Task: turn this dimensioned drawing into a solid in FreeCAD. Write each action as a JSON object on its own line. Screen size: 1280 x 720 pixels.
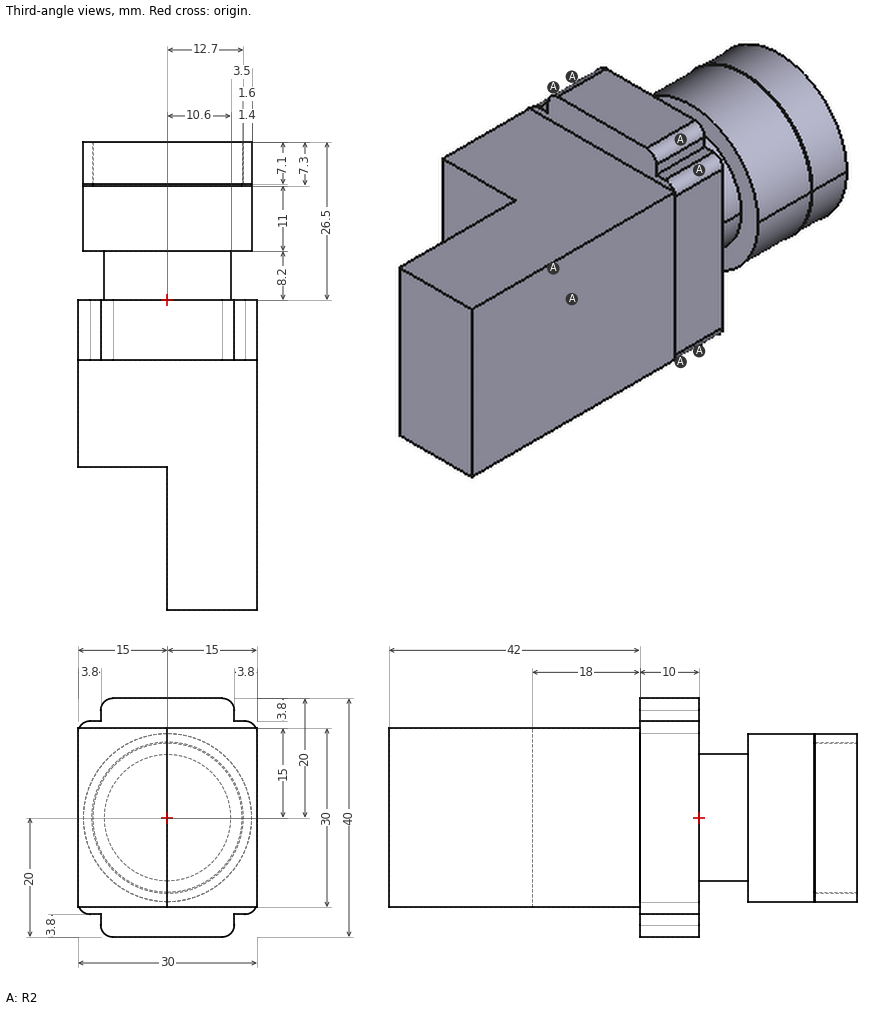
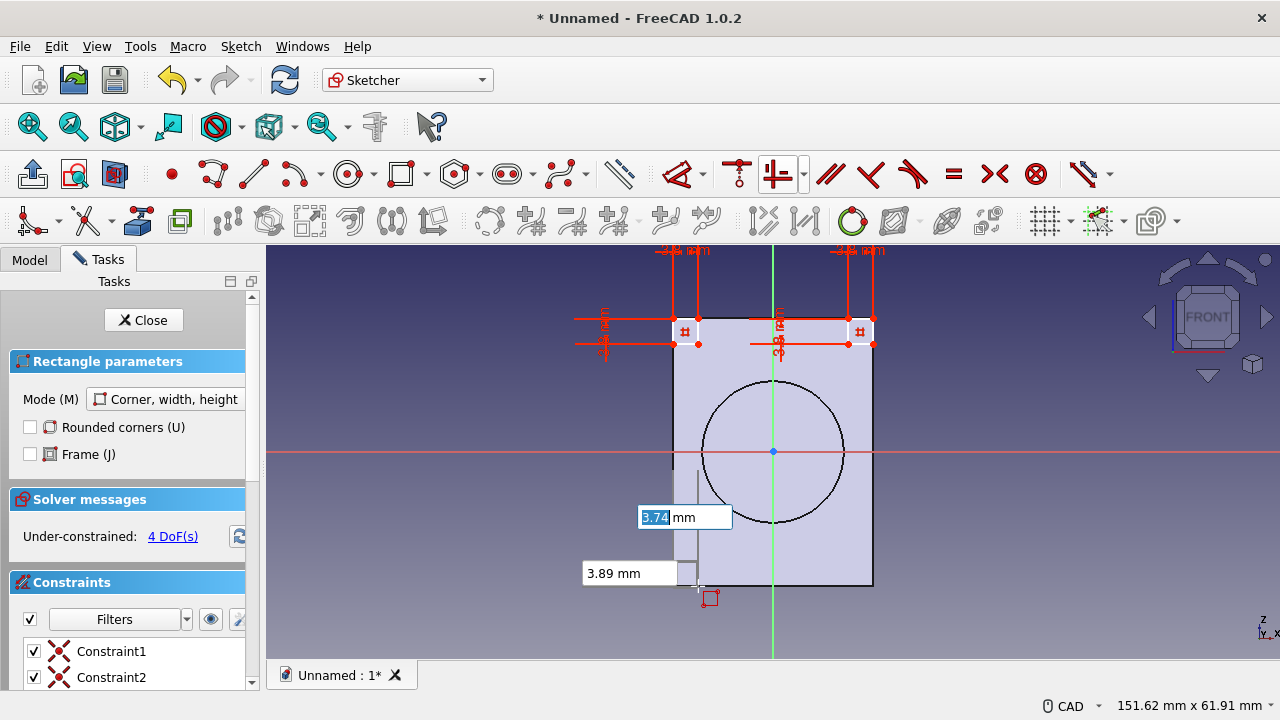
{"action": "type", "text": "3.8"}
{"action": "key", "text": "Tab"}
{"action": "type", "text": "3.8"}
{"action": "key", "text": "Return"}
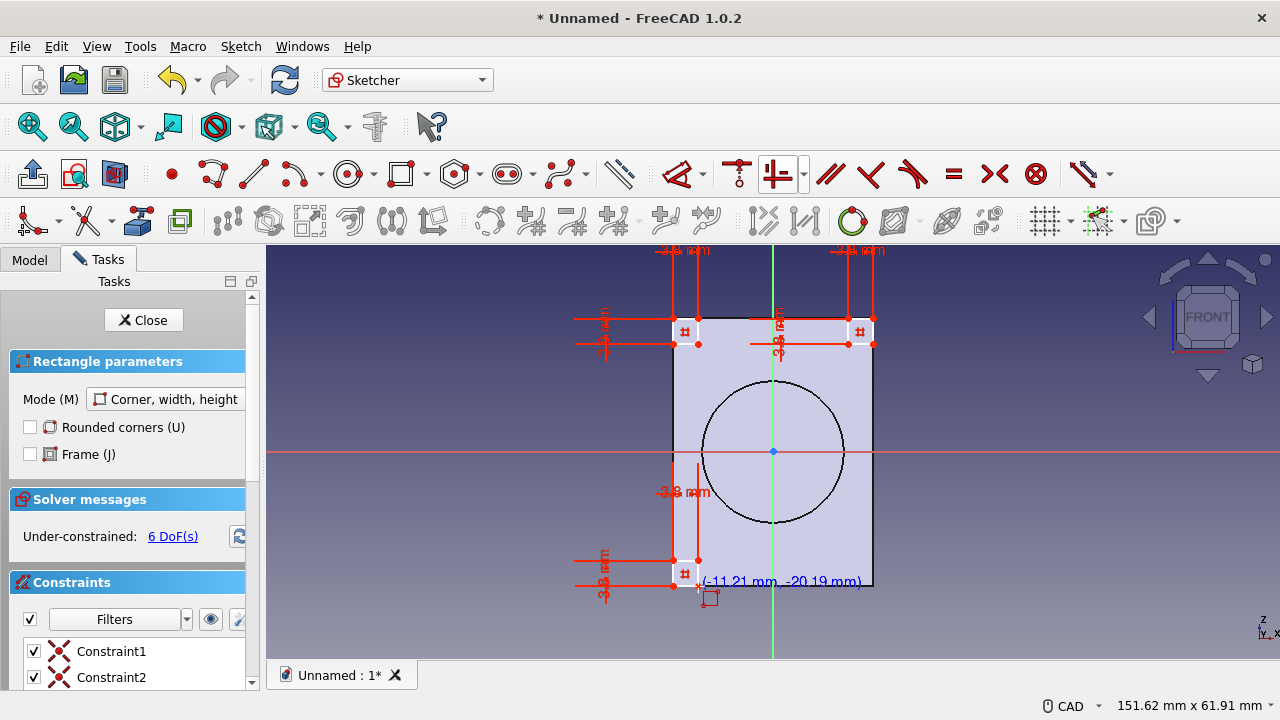
{"action": "left_click", "coordinate": [848, 560]}
{"action": "mouse_move", "coordinate": [873, 586]}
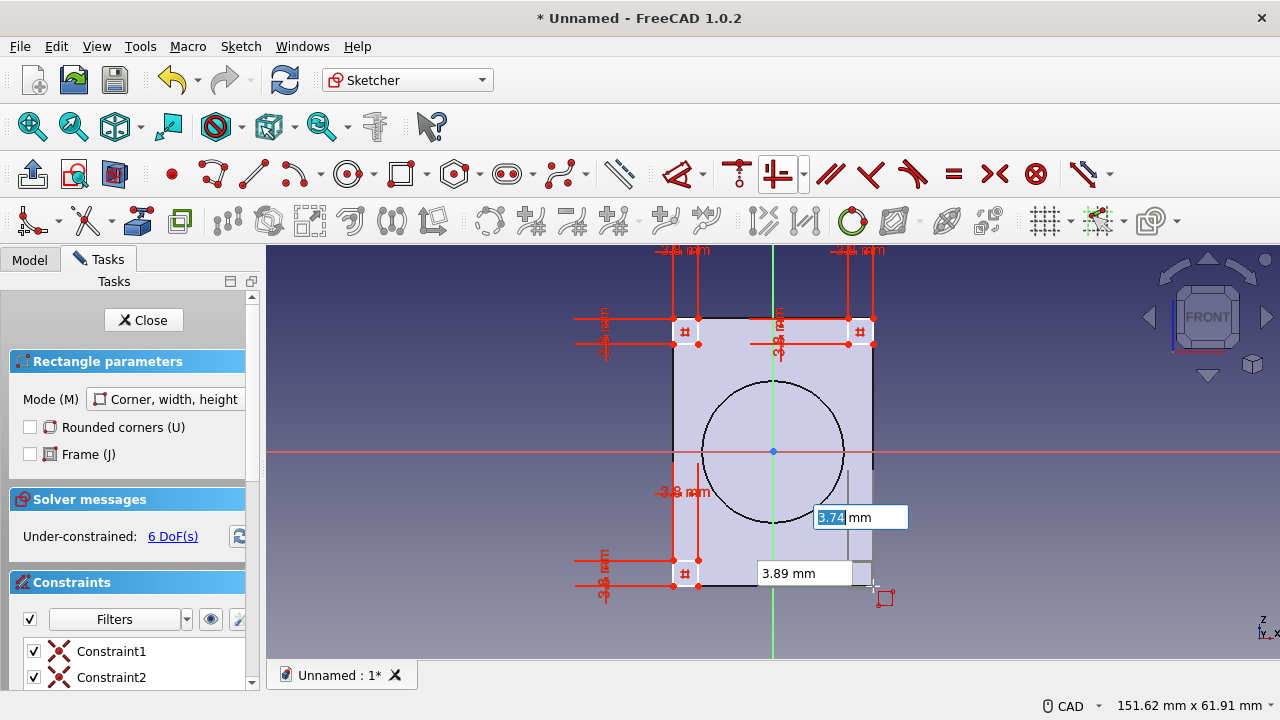
{"action": "type", "text": "3.8"}
{"action": "key", "text": "Tab"}
{"action": "type", "text": "3.8"}
{"action": "key", "text": "Return"}
{"action": "key", "text": "Escape"}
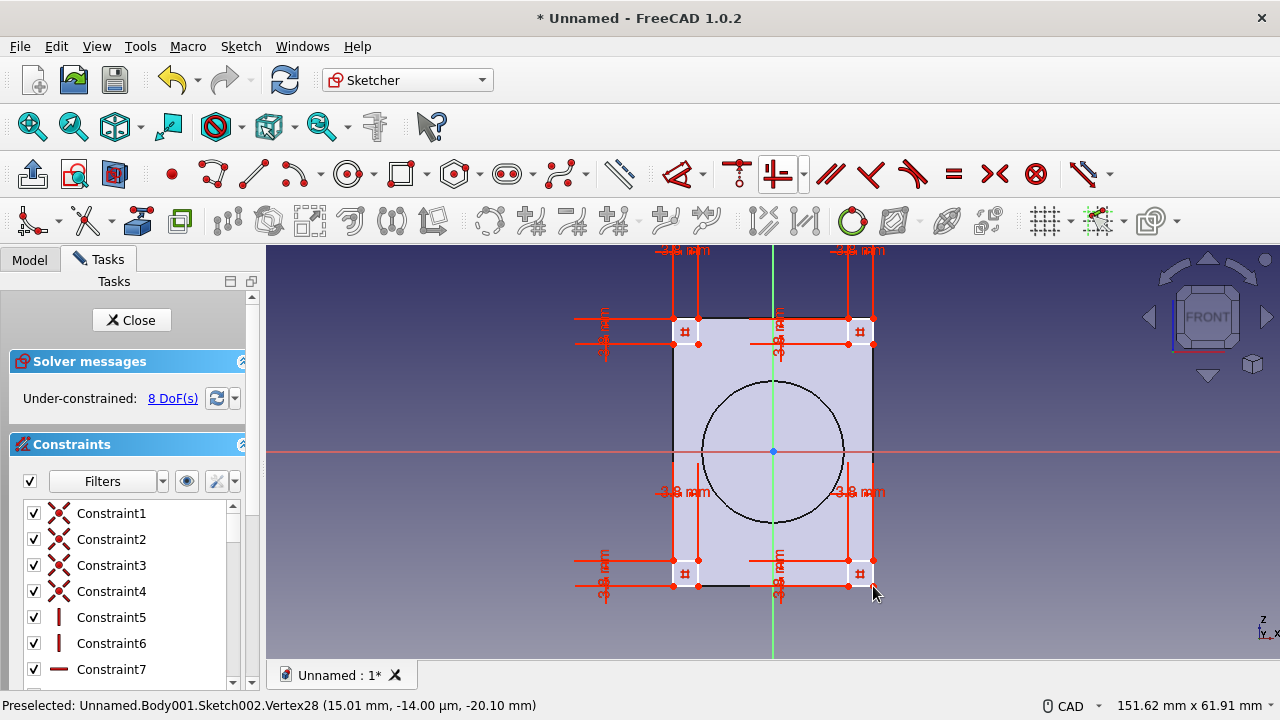
{"action": "key", "text": "d"}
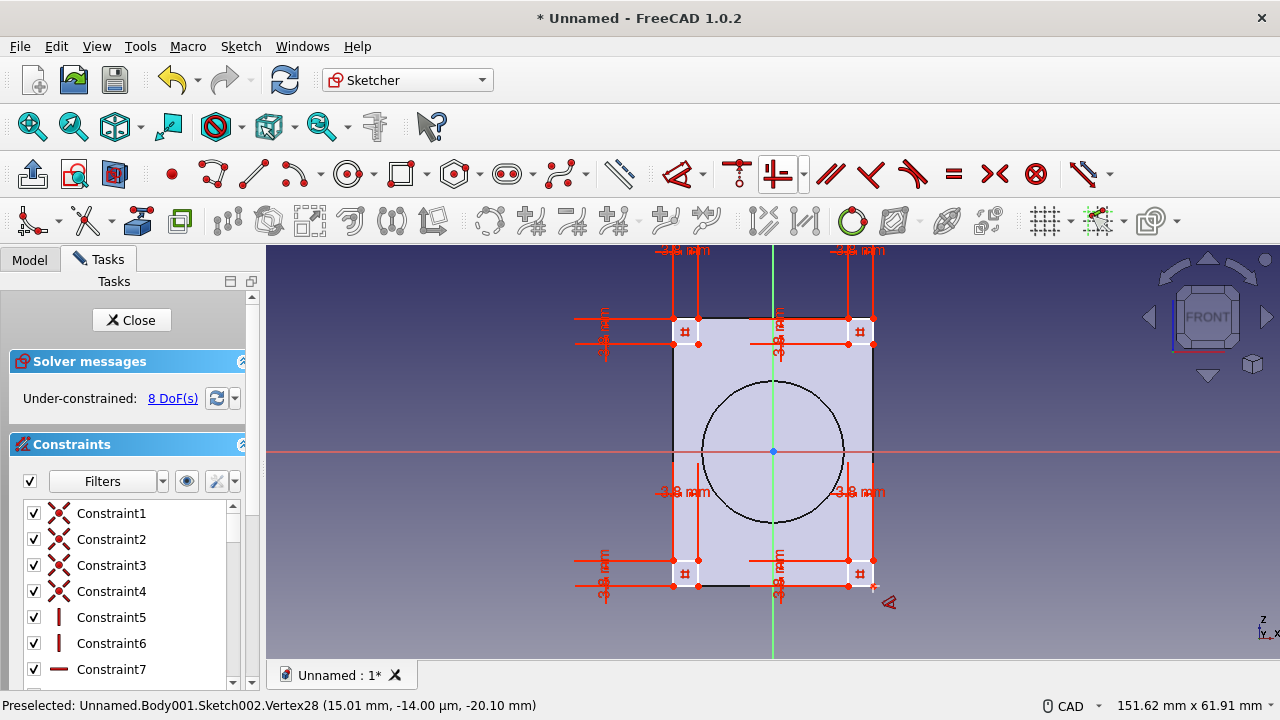
{"action": "left_click", "coordinate": [848, 319]}
{"action": "left_click", "coordinate": [882, 386]}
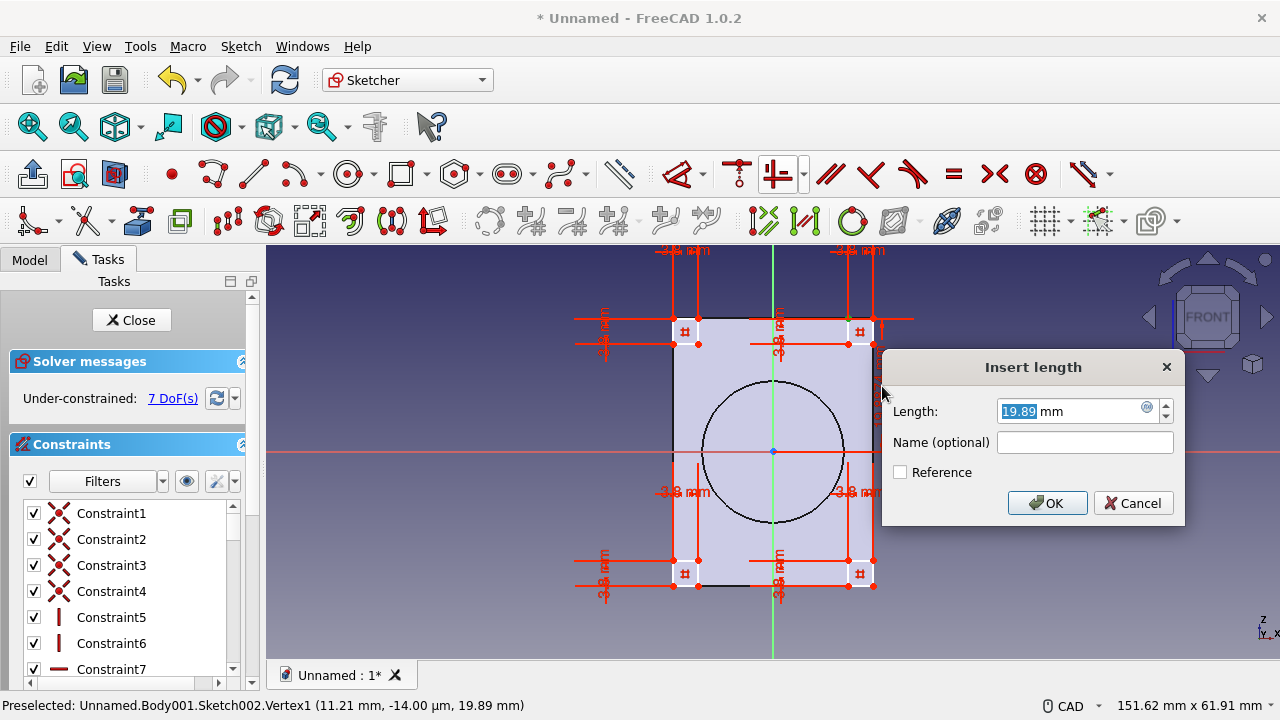
{"action": "type", "text": "20"}
{"action": "key", "text": "Return"}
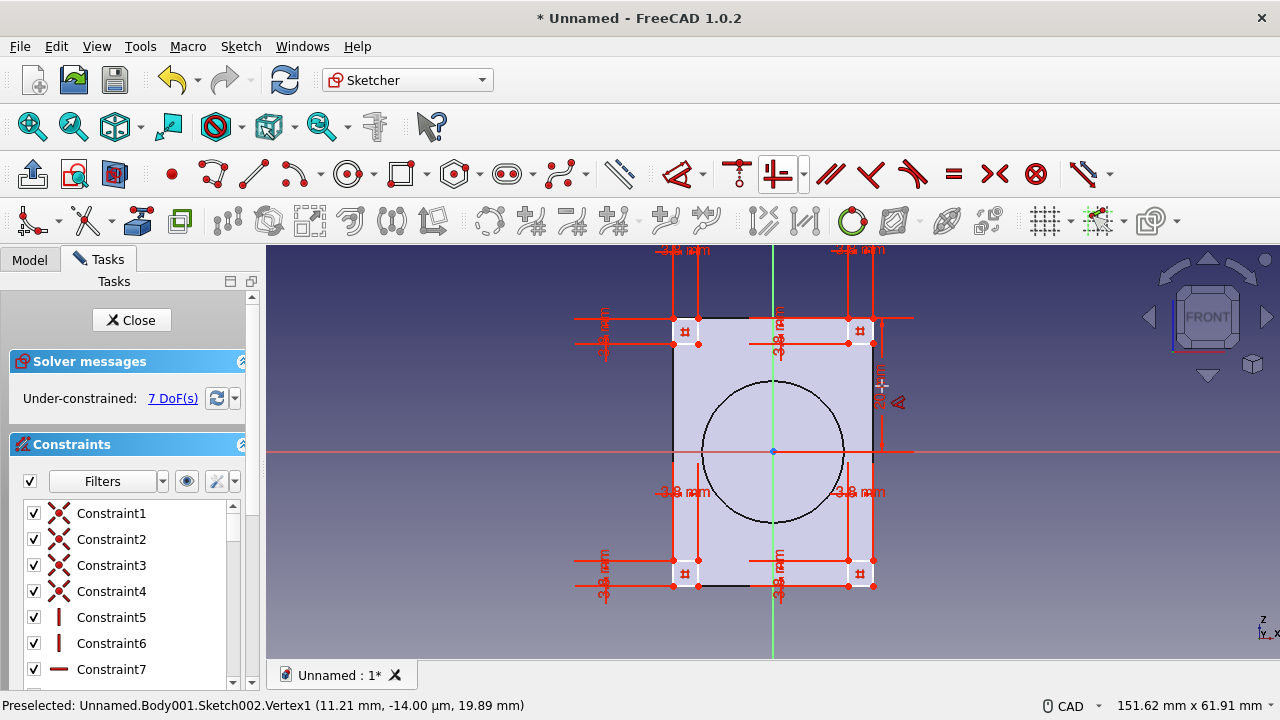
{"action": "left_click", "coordinate": [873, 344]}
{"action": "left_click", "coordinate": [823, 310]}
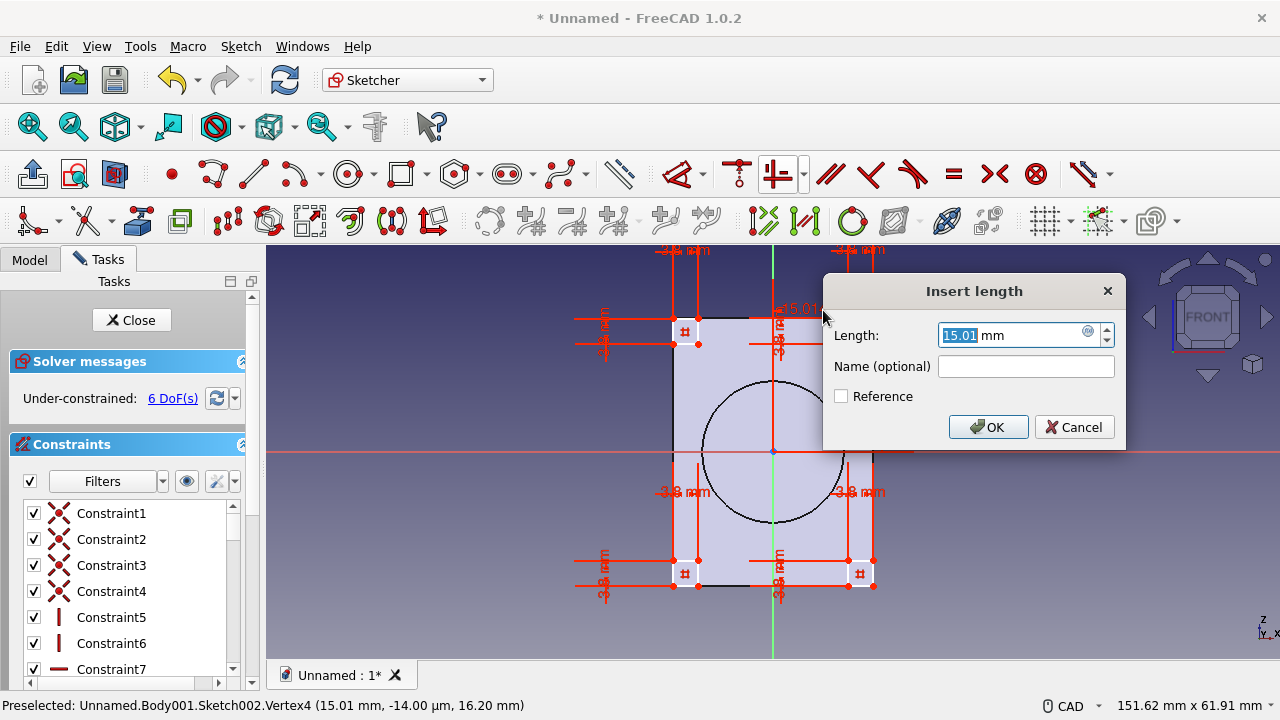
{"action": "type", "text": "15"}
{"action": "key", "text": "Return"}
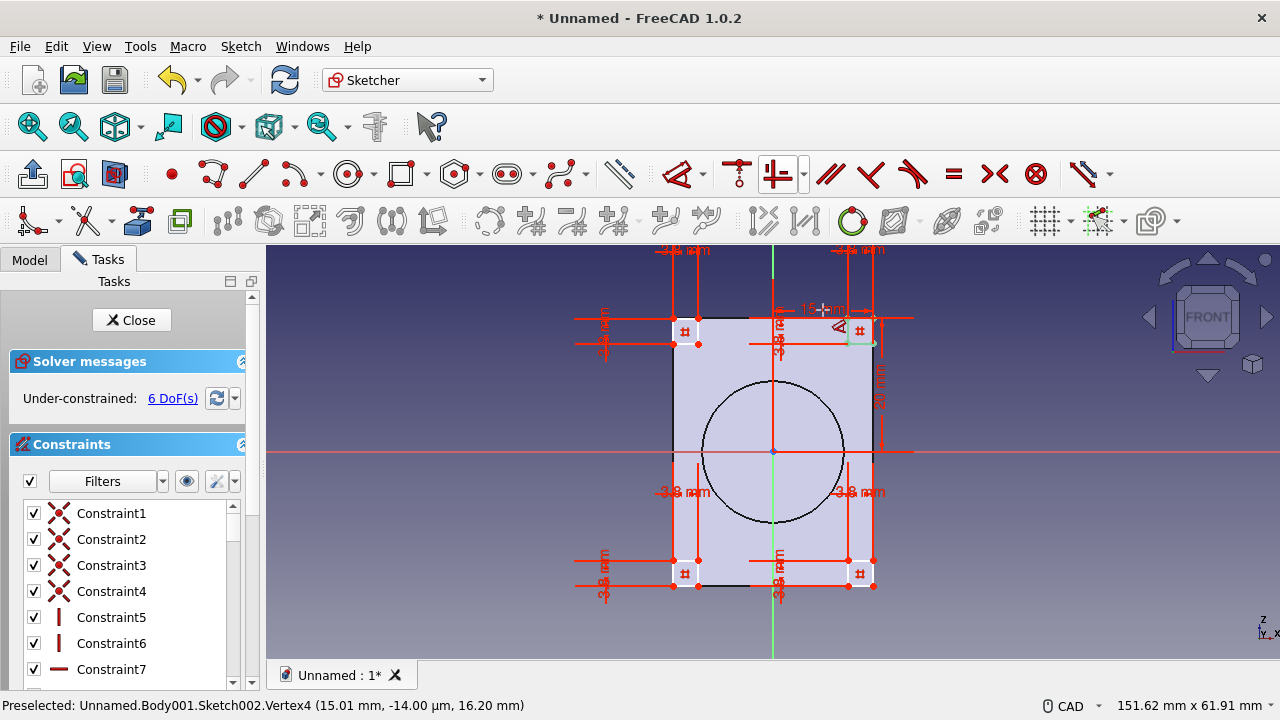
{"action": "left_click", "coordinate": [673, 319]}
{"action": "left_click", "coordinate": [723, 285]}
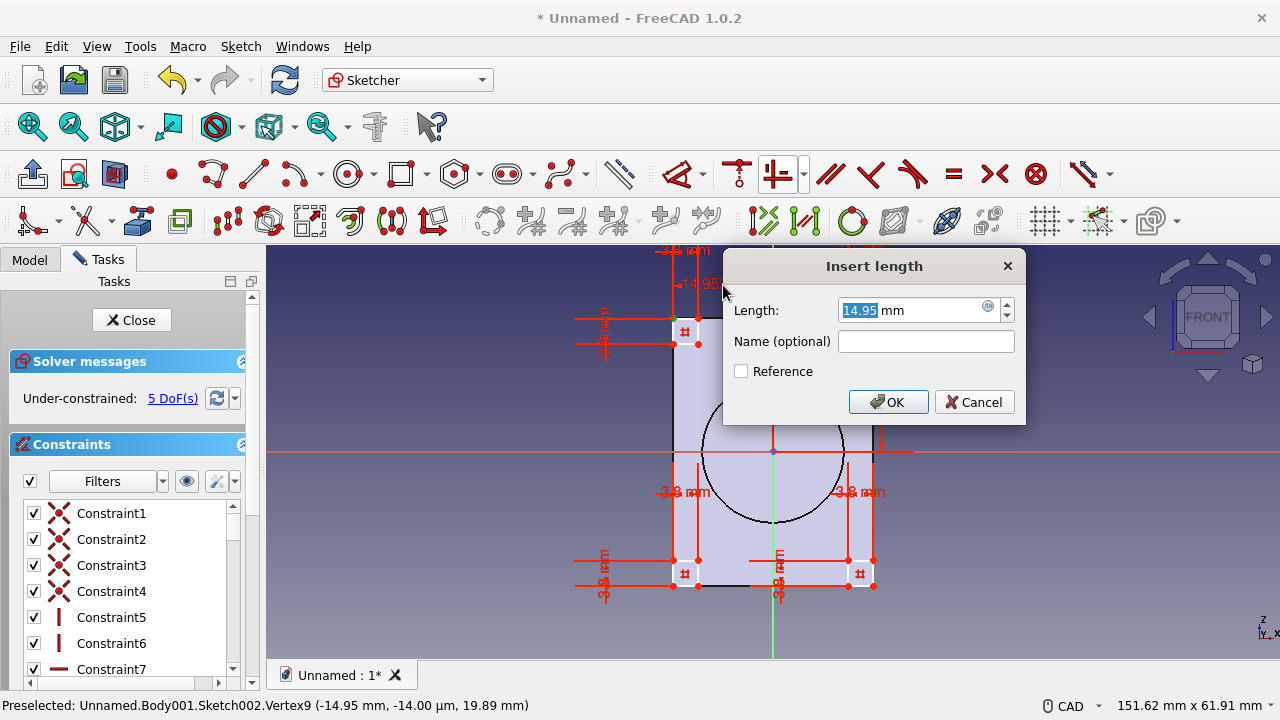
{"action": "type", "text": "15"}
{"action": "key", "text": "Return"}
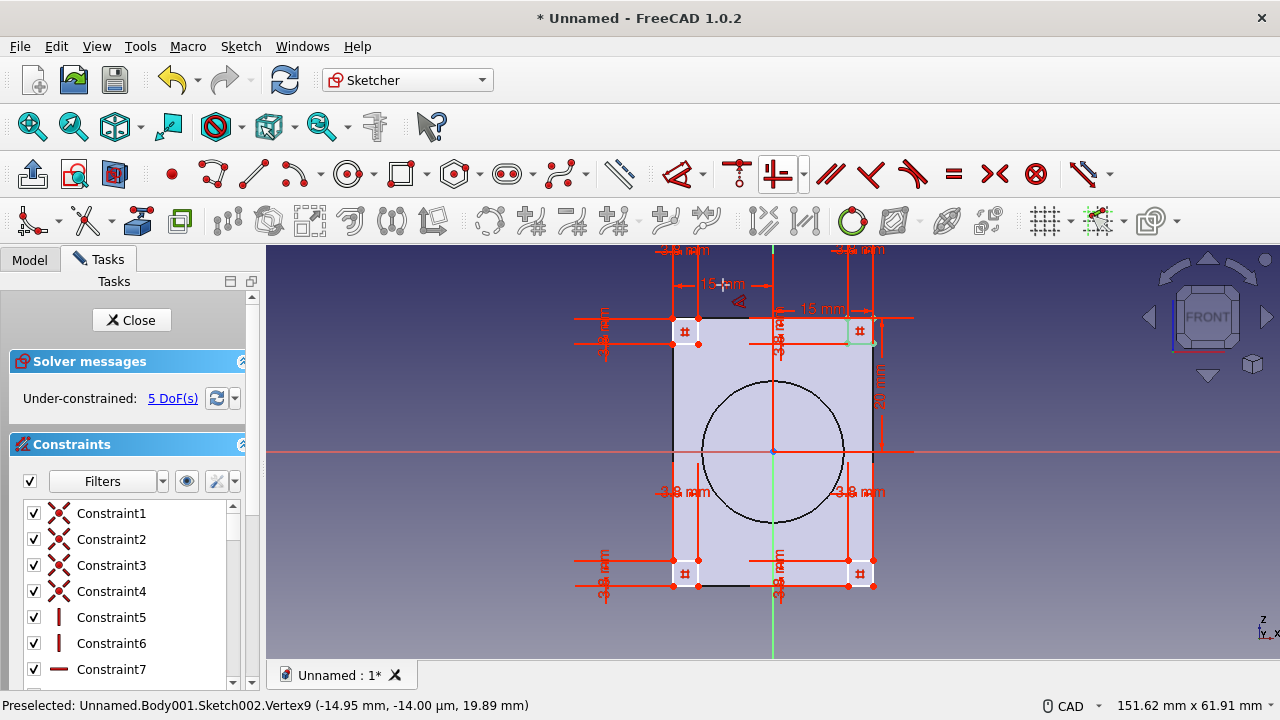
{"action": "left_click", "coordinate": [673, 319]}
{"action": "left_click", "coordinate": [639, 386]}